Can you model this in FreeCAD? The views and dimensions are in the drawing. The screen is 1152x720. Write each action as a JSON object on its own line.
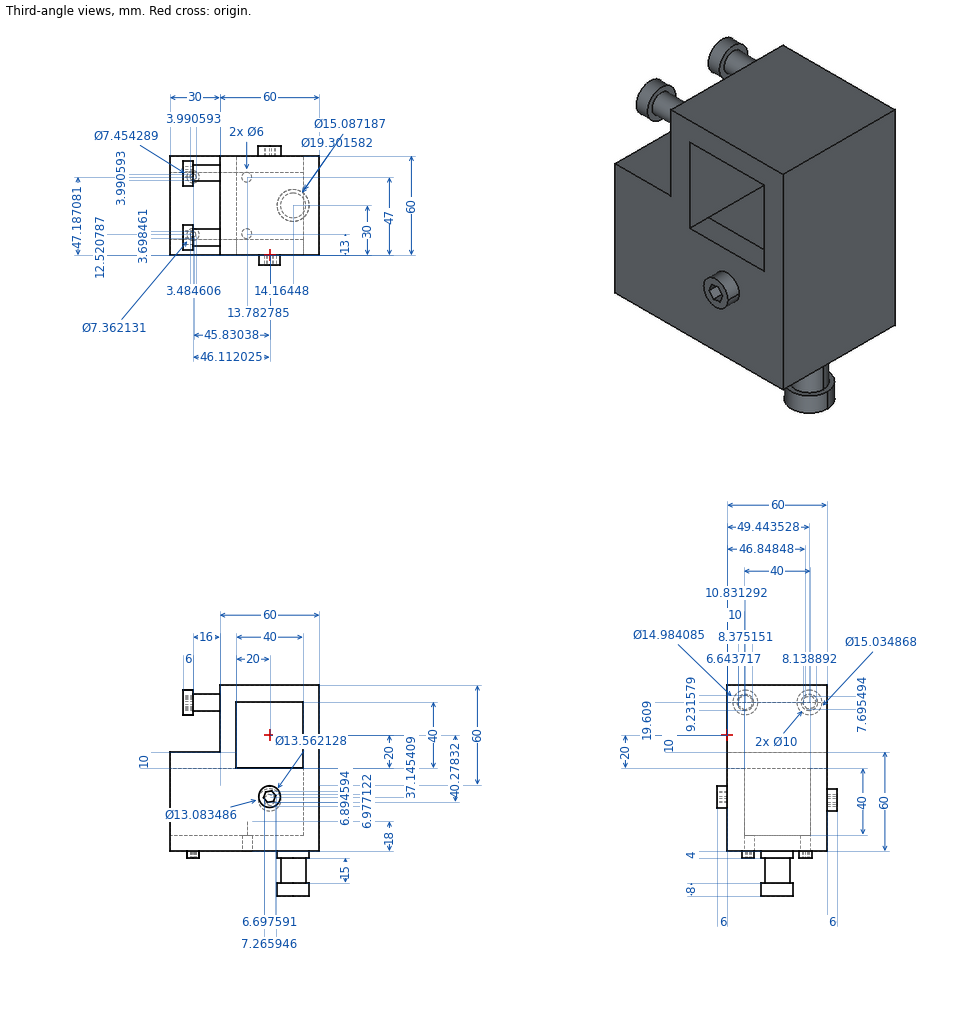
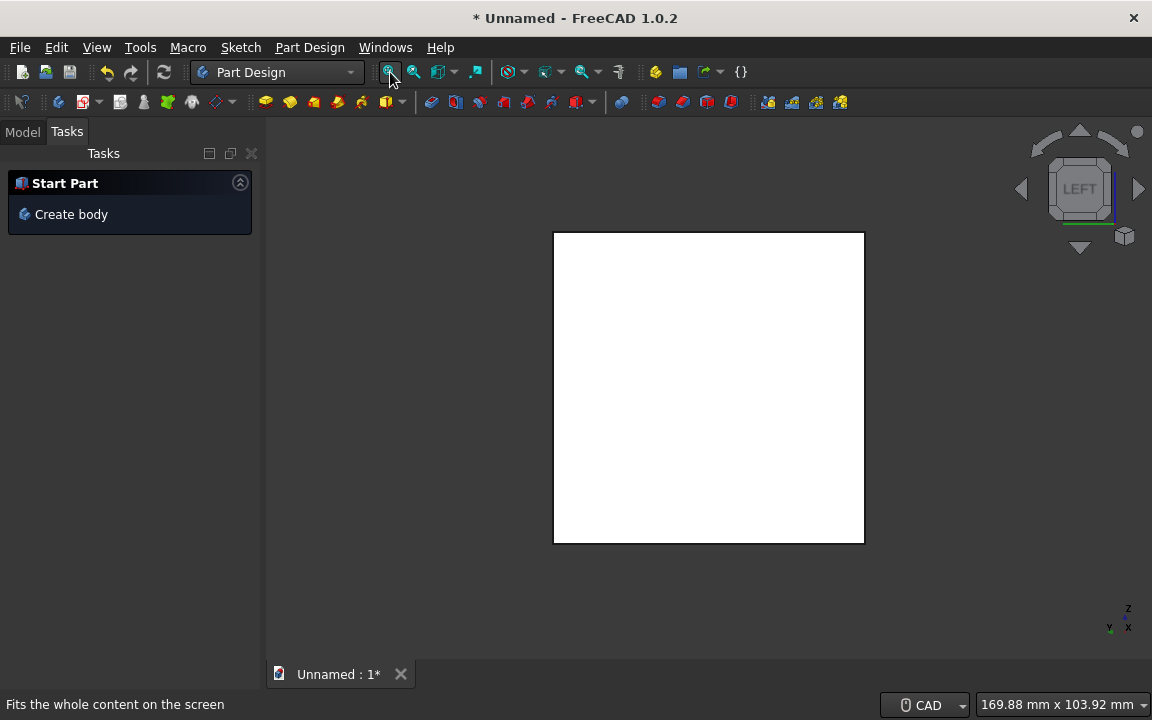
{"action": "left_click", "coordinate": [709, 387]}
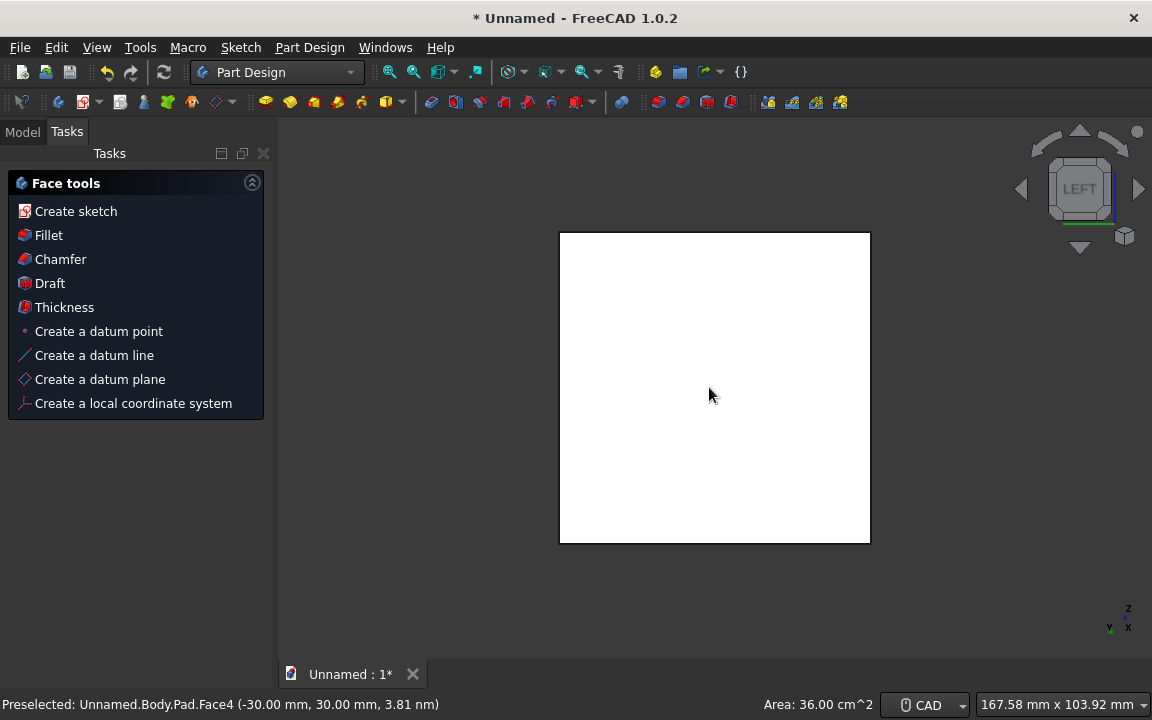
{"action": "left_click", "coordinate": [84, 102]}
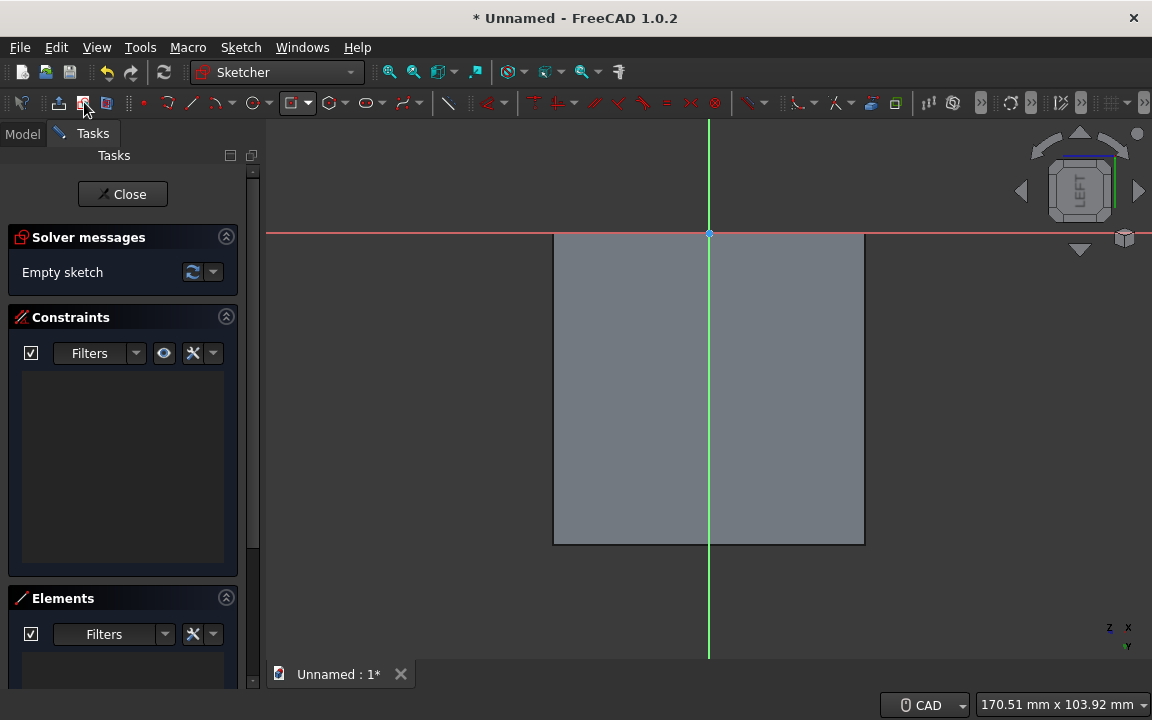
{"action": "scroll", "coordinate": [294, 389], "scroll_direction": "down", "scroll_amount": 1}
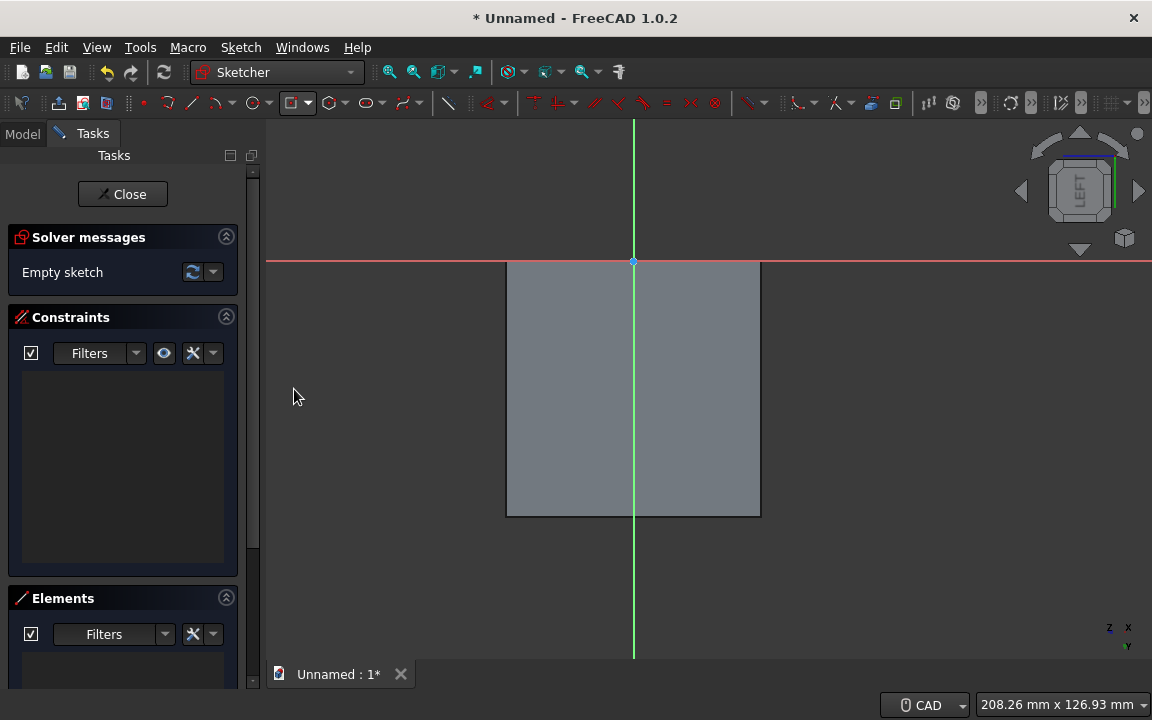
{"action": "key", "text": "g r"}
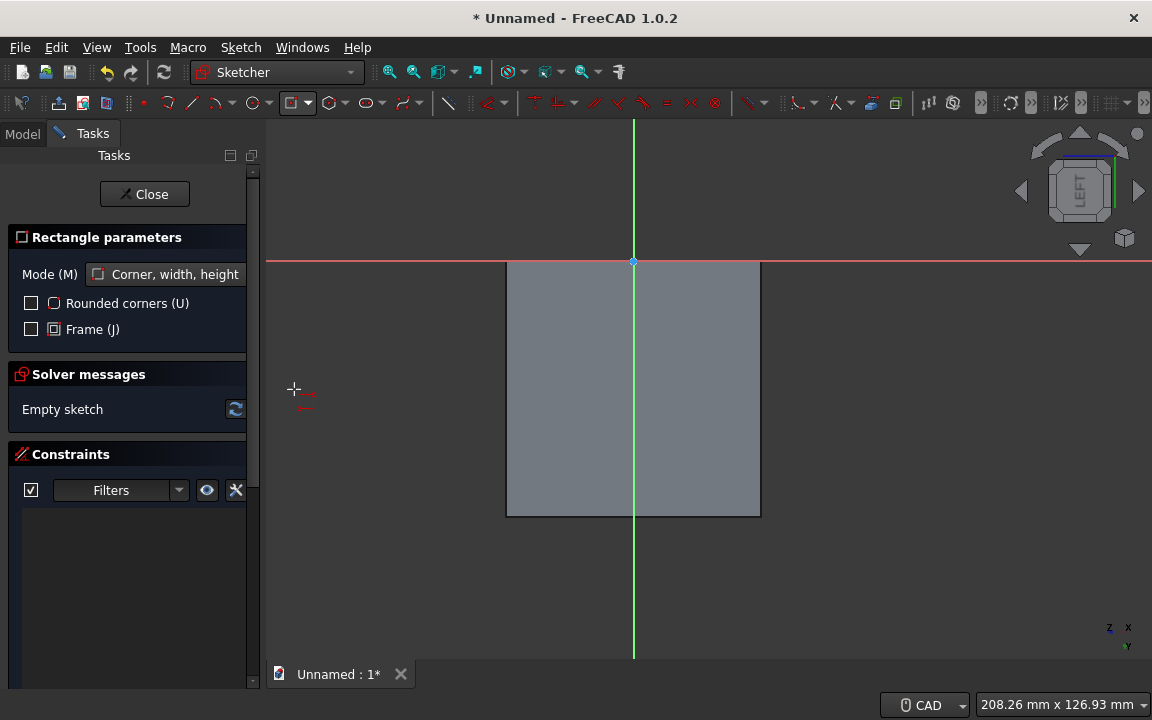
{"action": "left_click", "coordinate": [676, 261]}
{"action": "left_click", "coordinate": [932, 517]}
{"action": "key", "text": "Escape"}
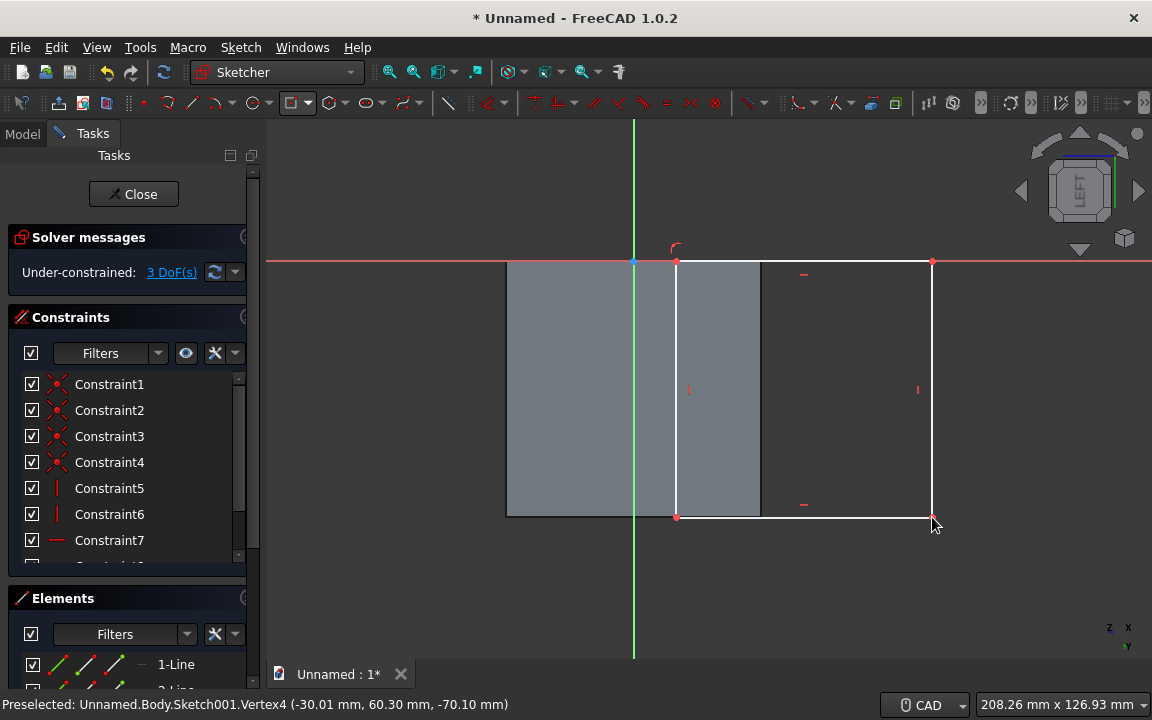
{"action": "left_click", "coordinate": [488, 104]}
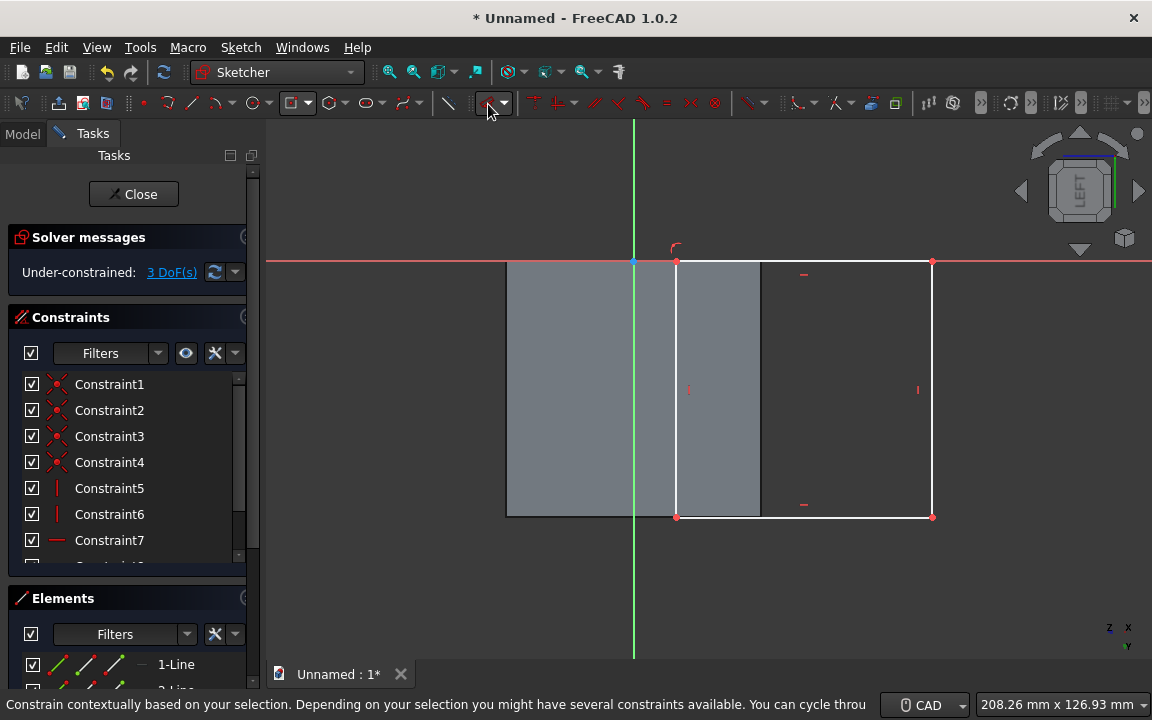
{"action": "left_click", "coordinate": [676, 338]}
{"action": "left_click", "coordinate": [710, 390]}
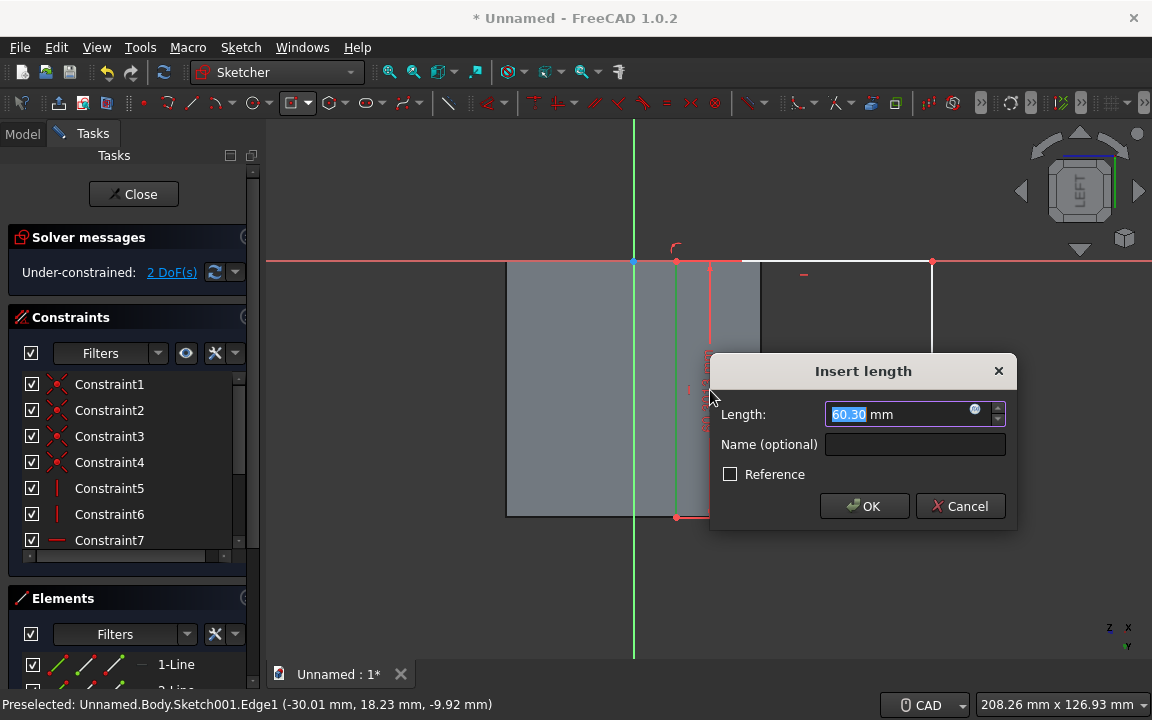
{"action": "type", "text": "60"}
{"action": "key", "text": "Return"}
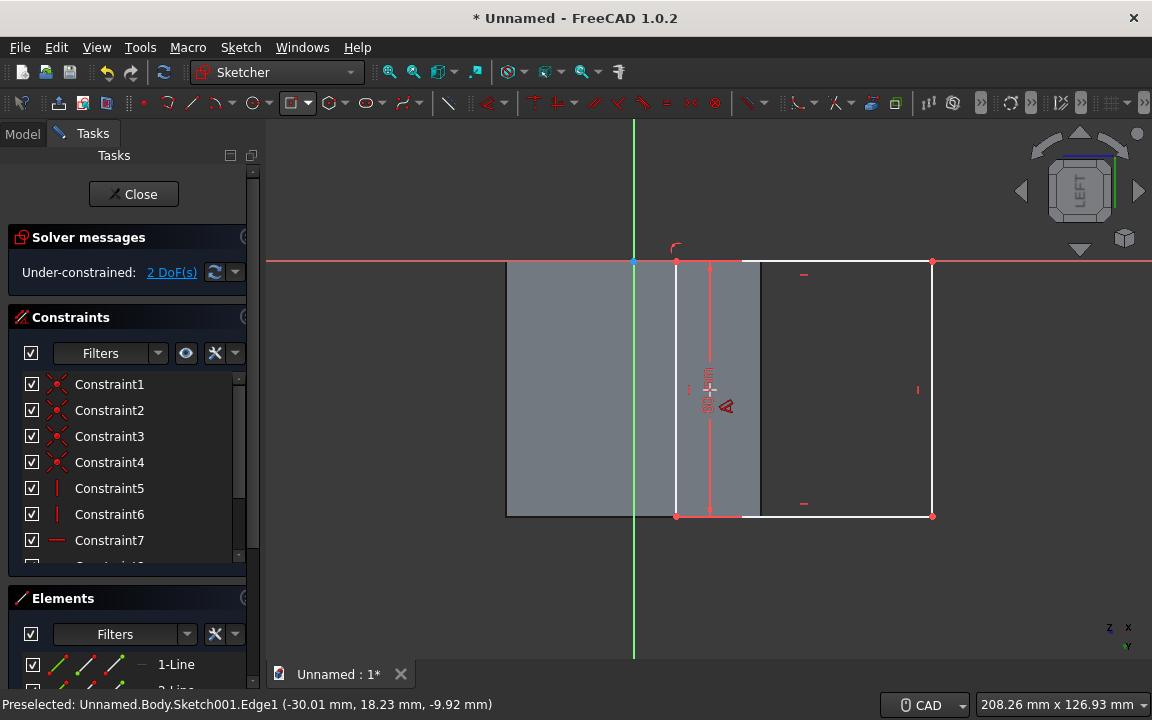
{"action": "left_click", "coordinate": [753, 517]}
{"action": "left_click", "coordinate": [804, 551]}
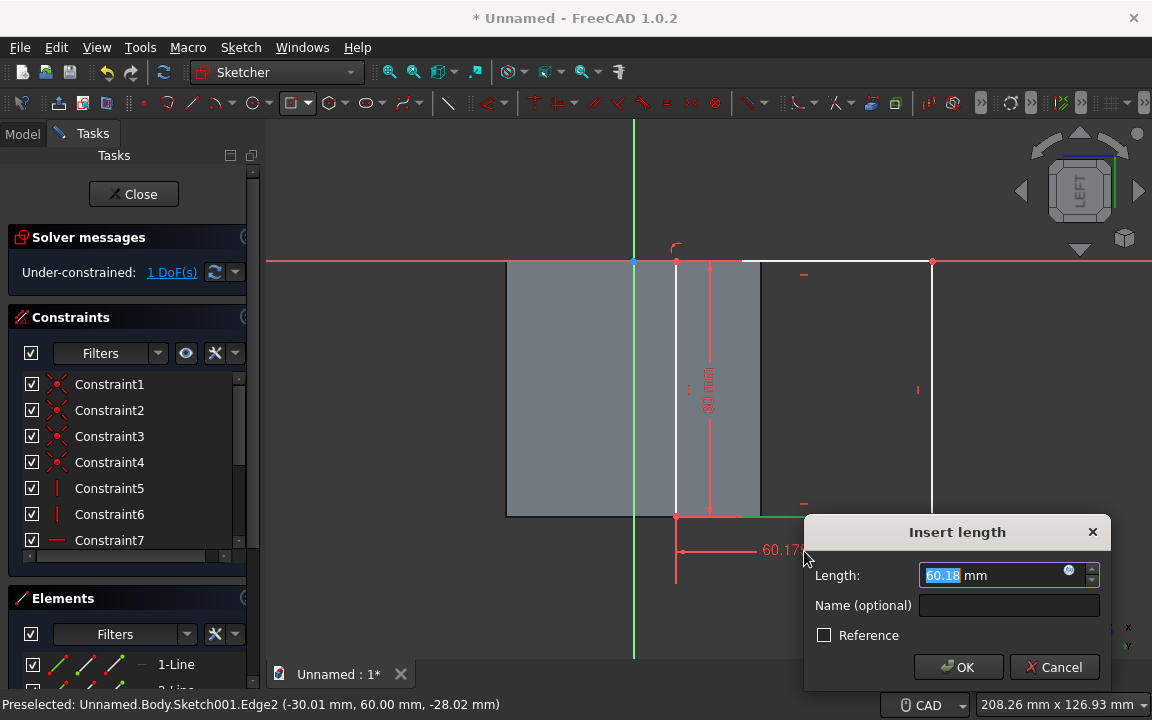
{"action": "type", "text": "60"}
{"action": "key", "text": "Return"}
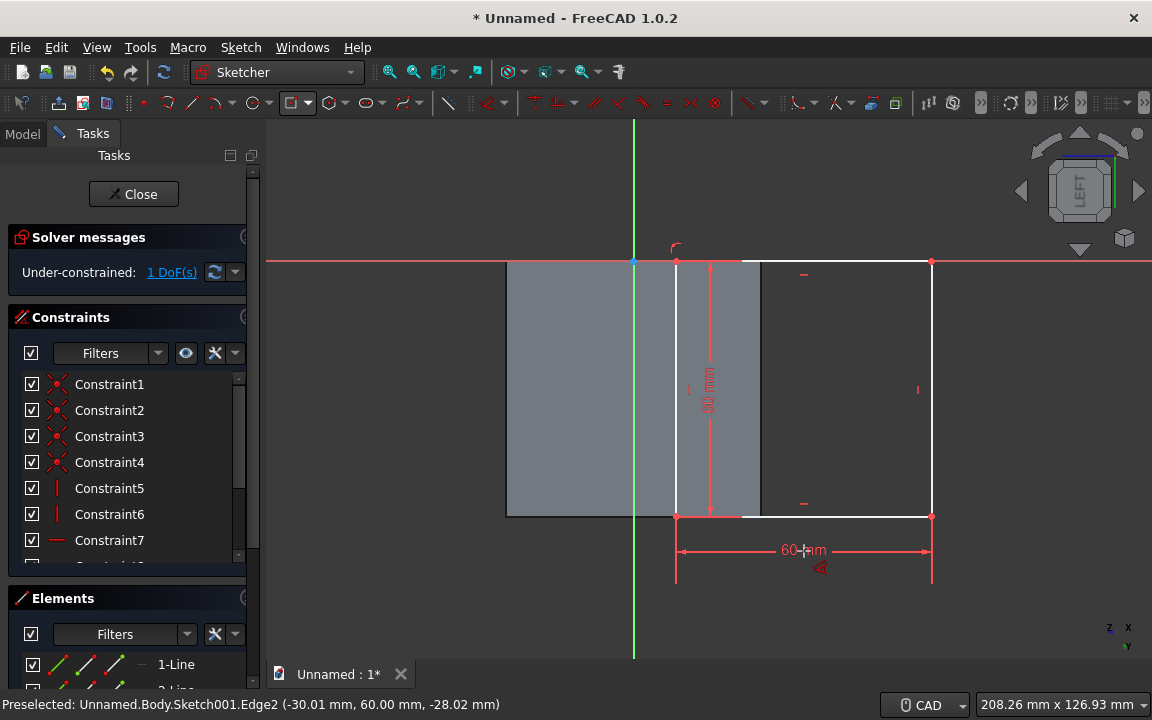
{"action": "left_click", "coordinate": [676, 261]}
{"action": "left_click", "coordinate": [655, 227]}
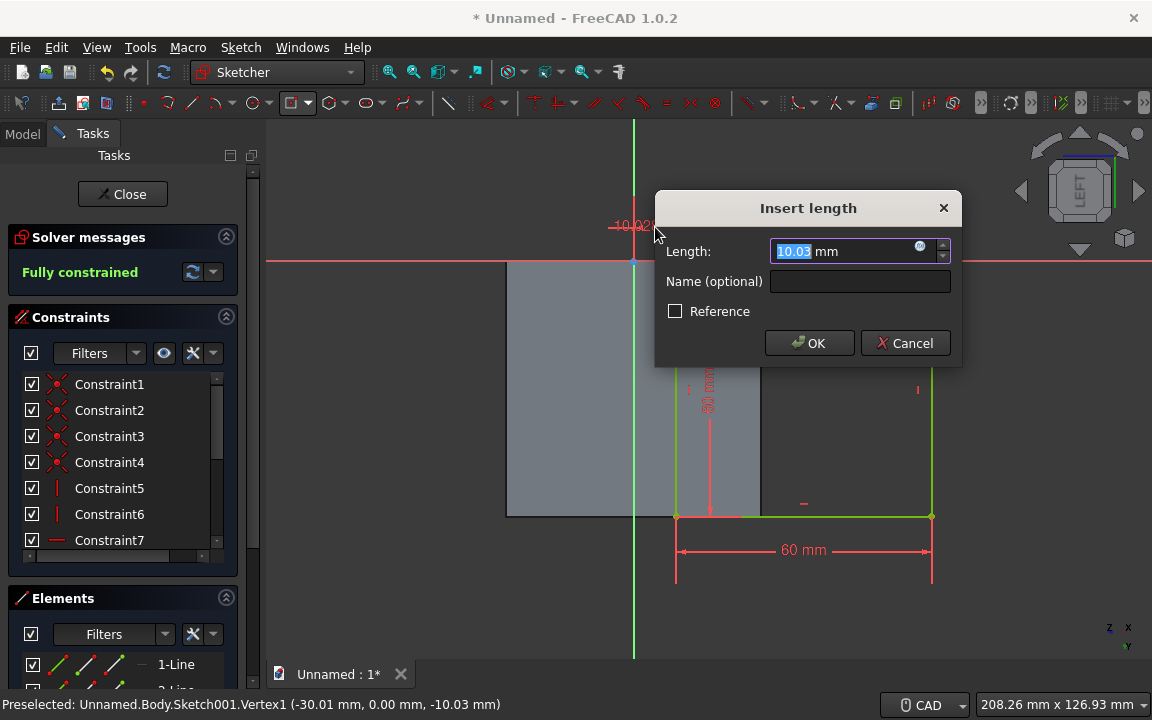
{"action": "type", "text": "10"}
{"action": "key", "text": "Return"}
{"action": "key", "text": "Escape"}